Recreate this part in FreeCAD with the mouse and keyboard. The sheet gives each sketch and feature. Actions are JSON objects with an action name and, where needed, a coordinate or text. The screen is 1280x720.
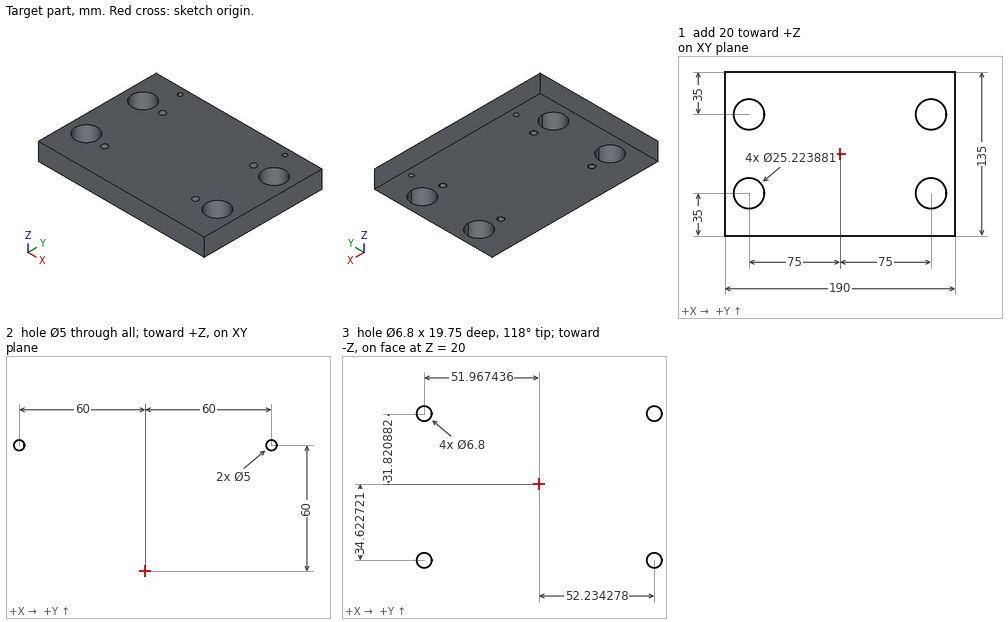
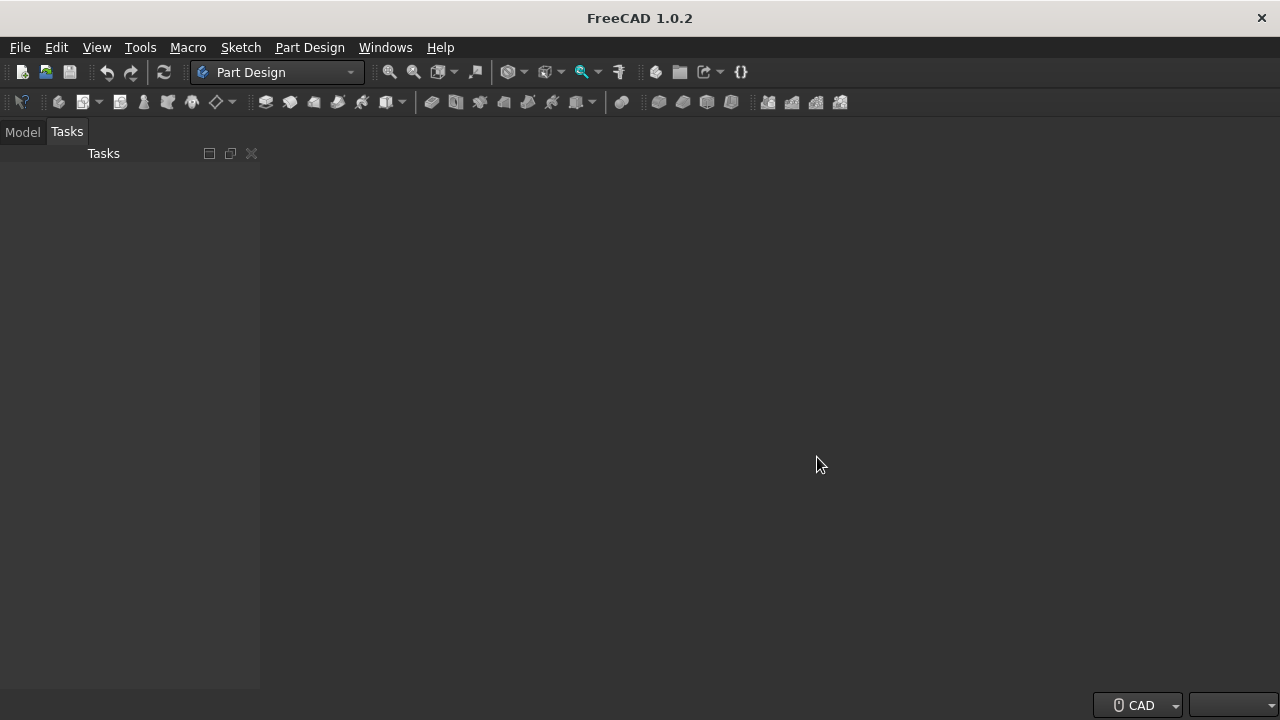
{"action": "left_click", "coordinate": [22, 72]}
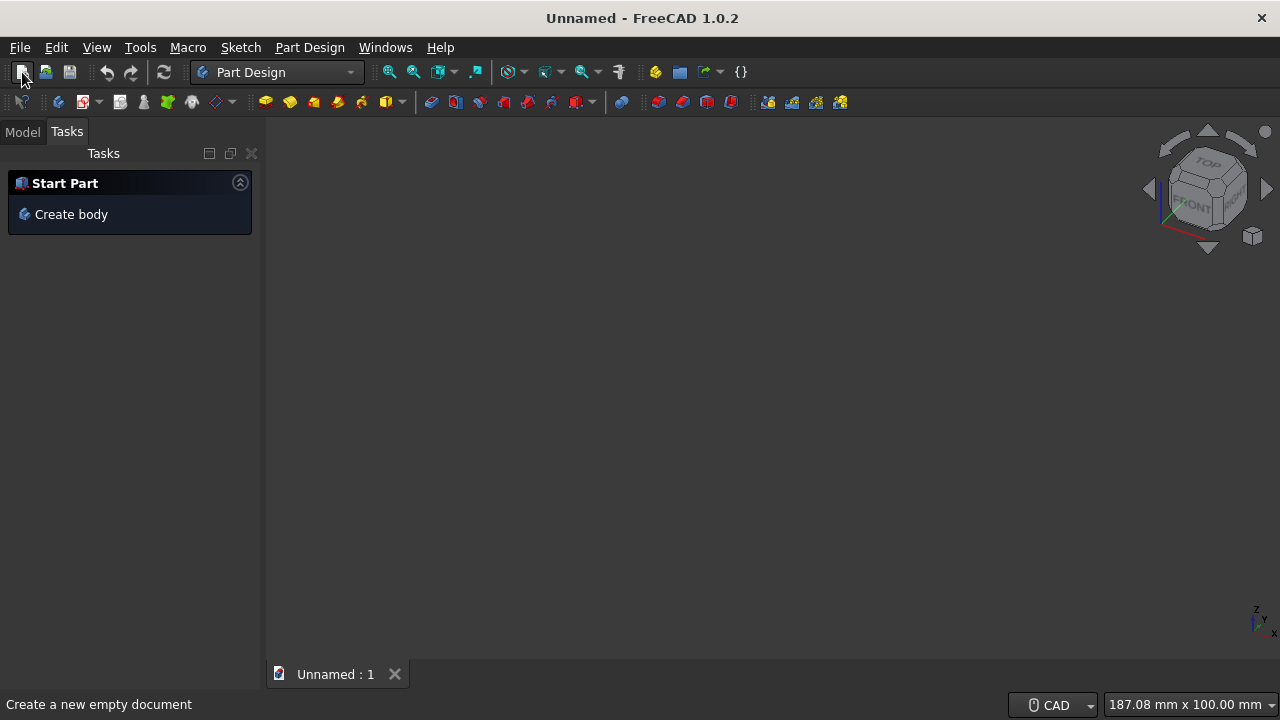
{"action": "left_click", "coordinate": [84, 102]}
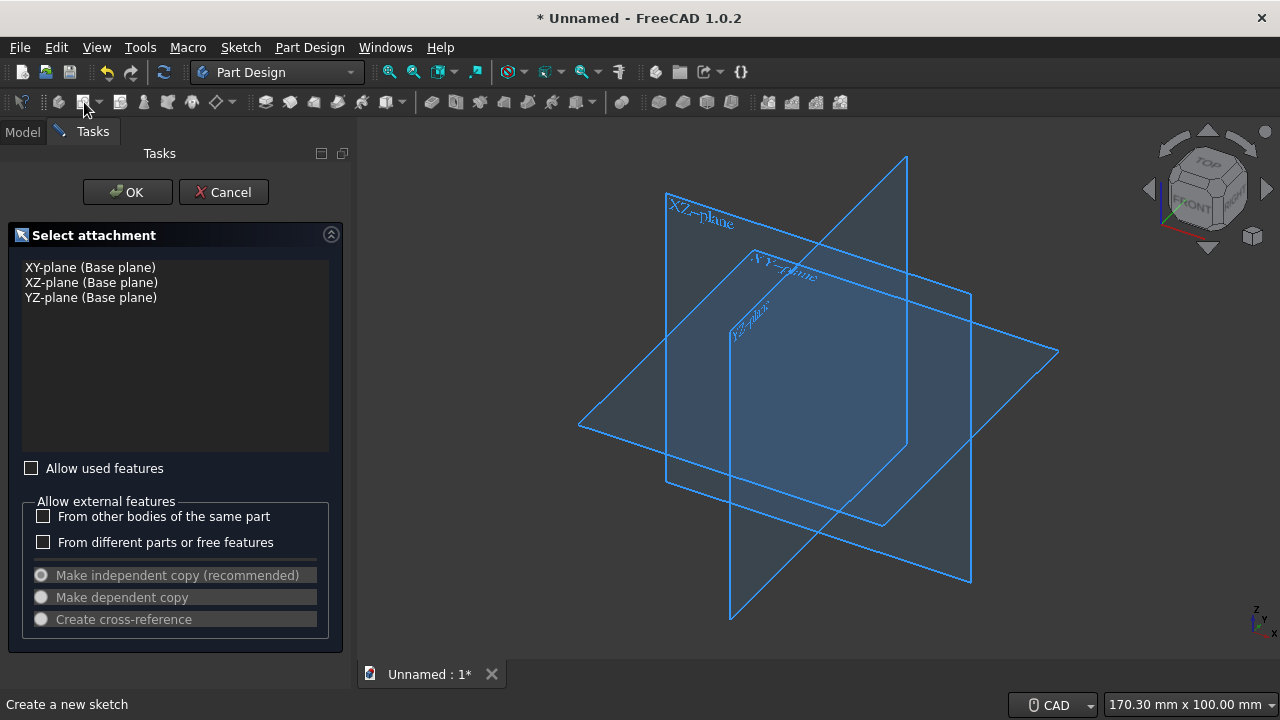
{"action": "left_click", "coordinate": [82, 268]}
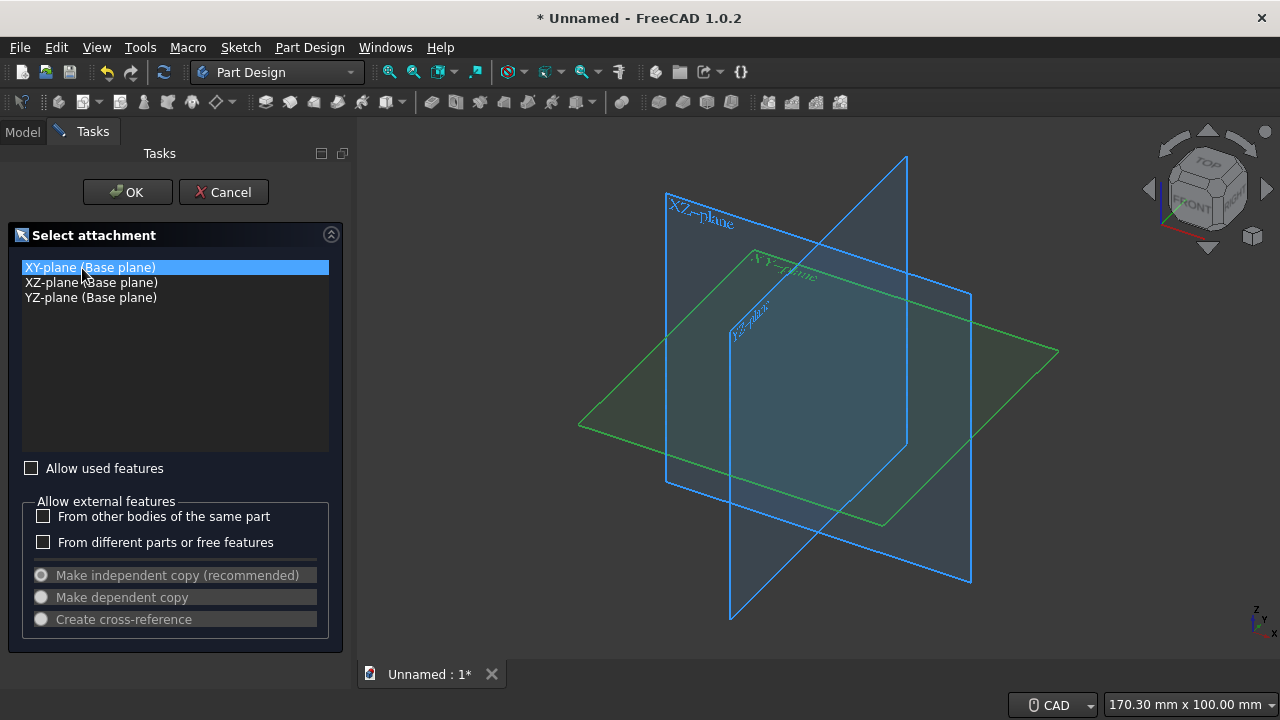
{"action": "left_click", "coordinate": [128, 192]}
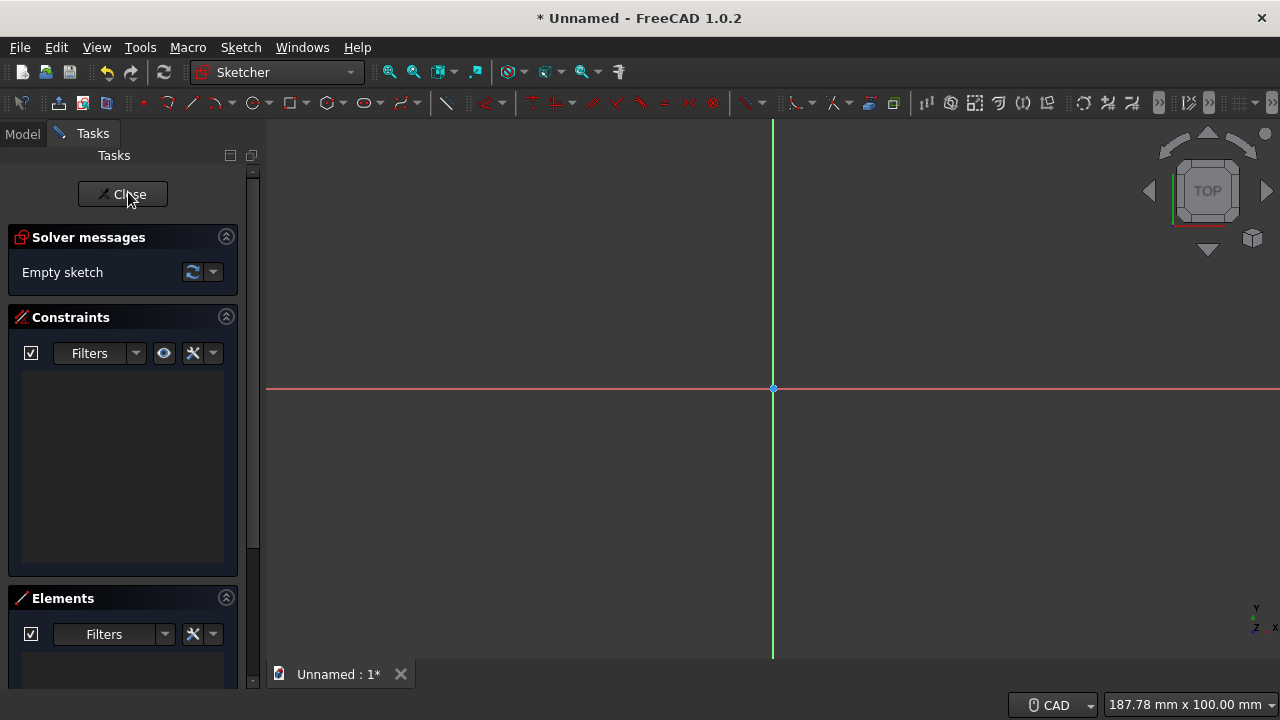
{"action": "scroll", "coordinate": [649, 389], "scroll_direction": "down", "scroll_amount": 4}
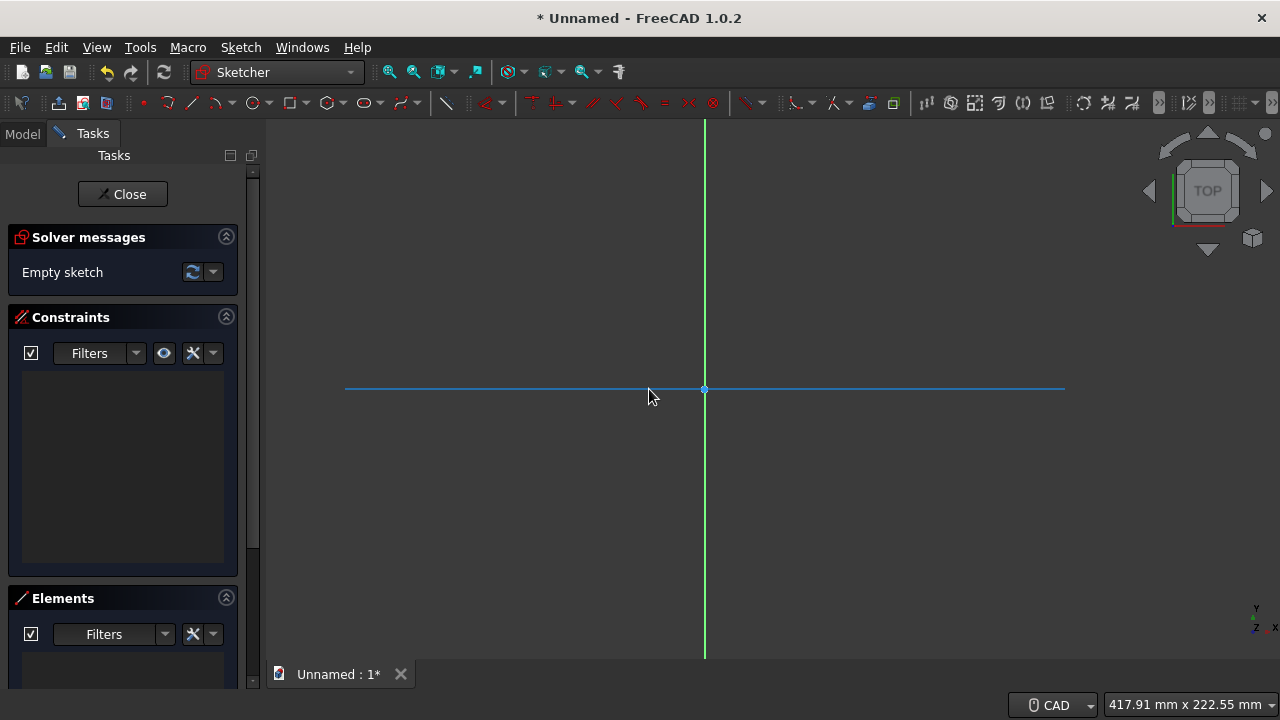
{"action": "left_click", "coordinate": [308, 104]}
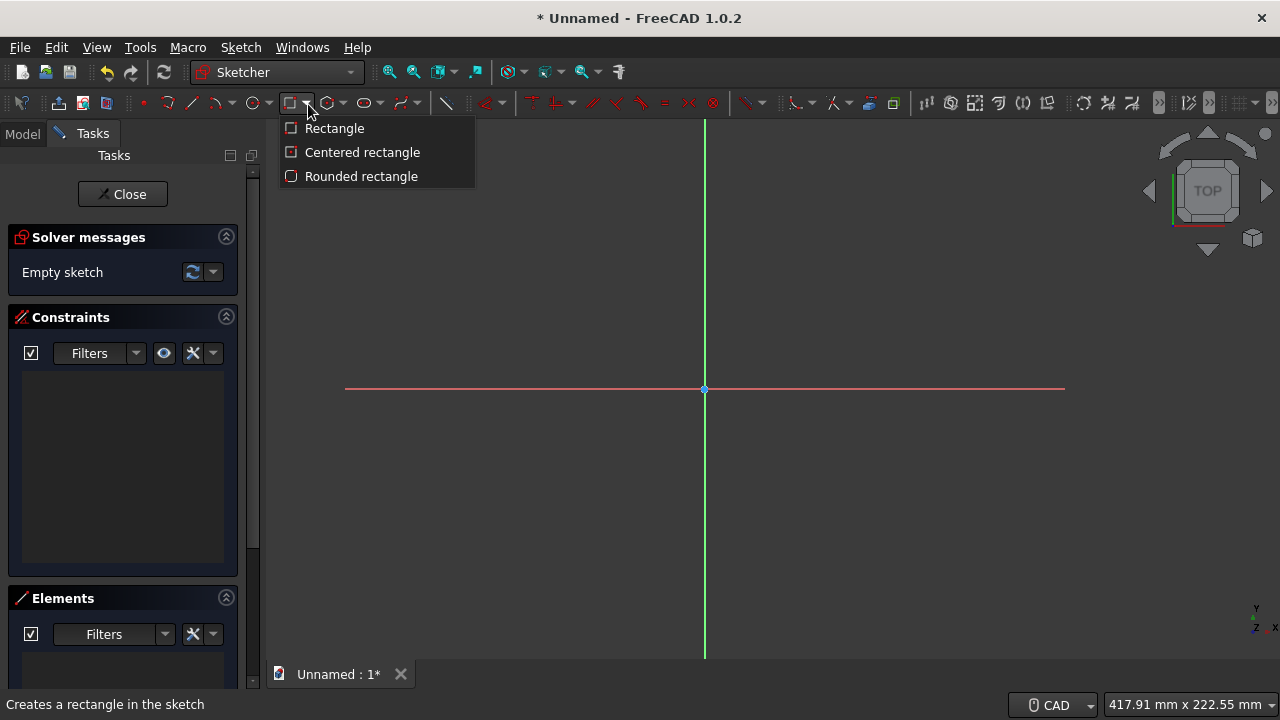
{"action": "left_click", "coordinate": [378, 152]}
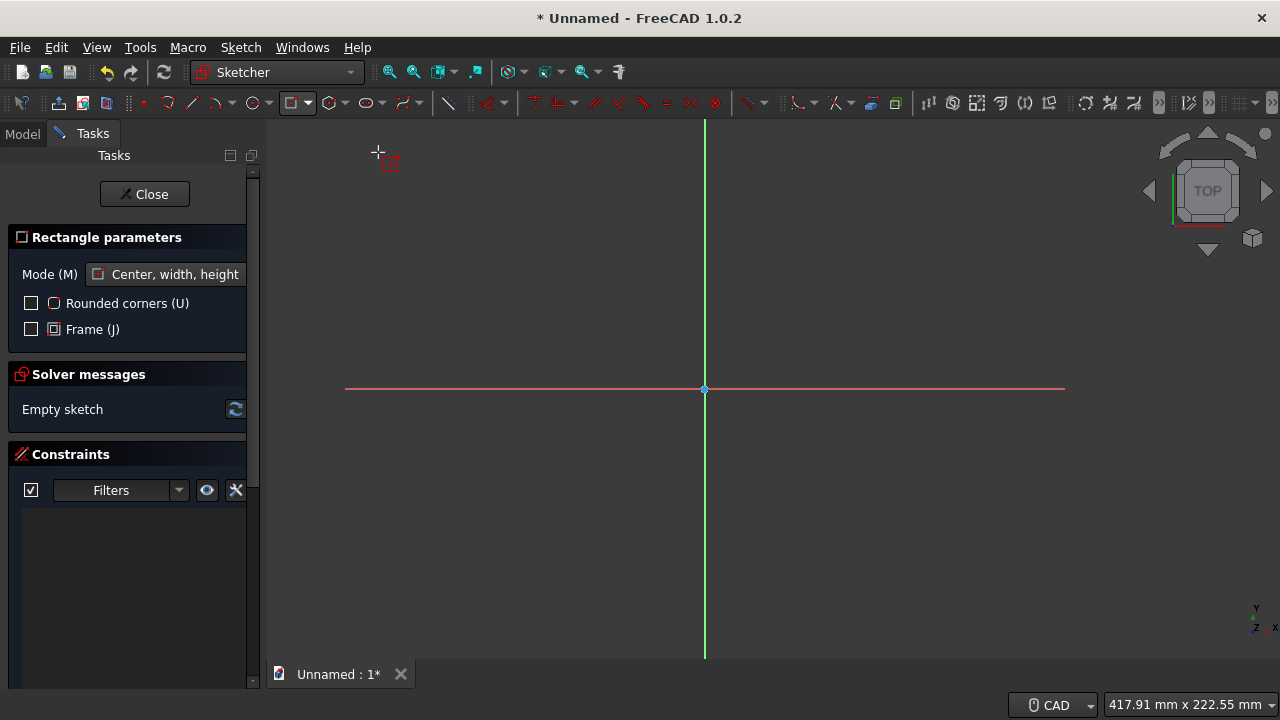
{"action": "left_click", "coordinate": [705, 389]}
{"action": "mouse_move", "coordinate": [935, 225]}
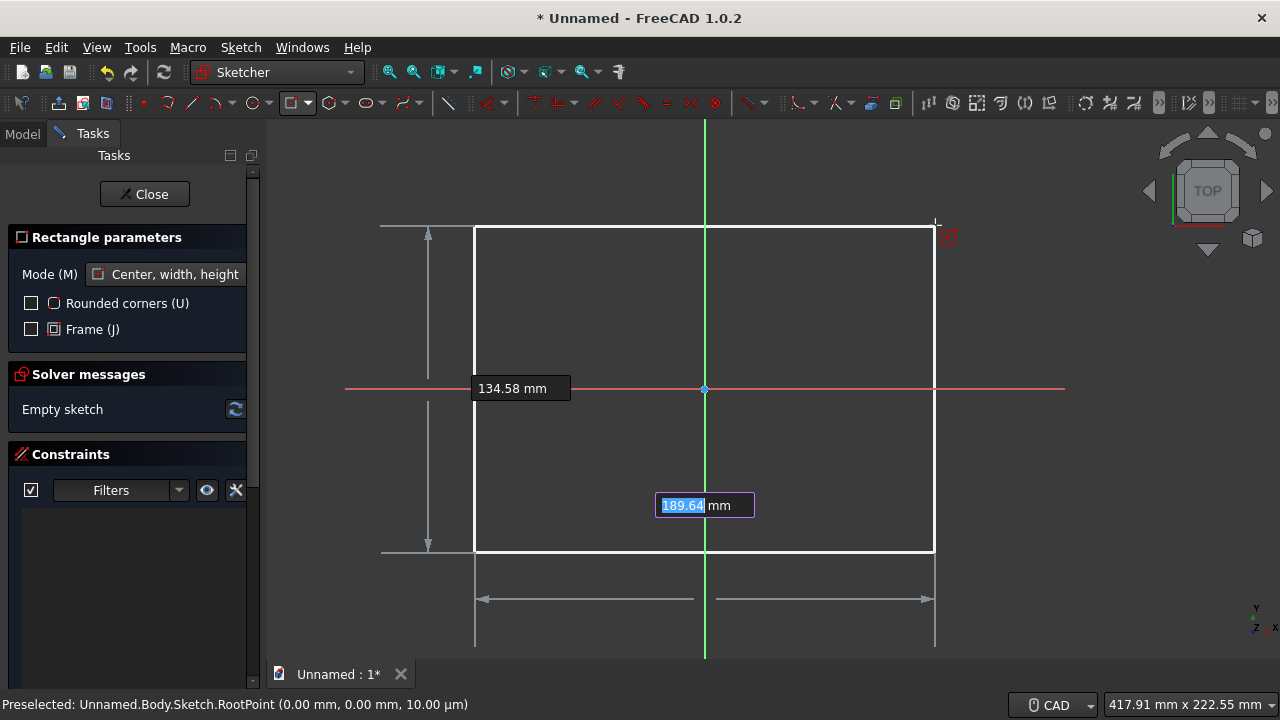
{"action": "type", "text": "190"}
{"action": "key", "text": "Tab"}
{"action": "type", "text": "135"}
{"action": "key", "text": "Return"}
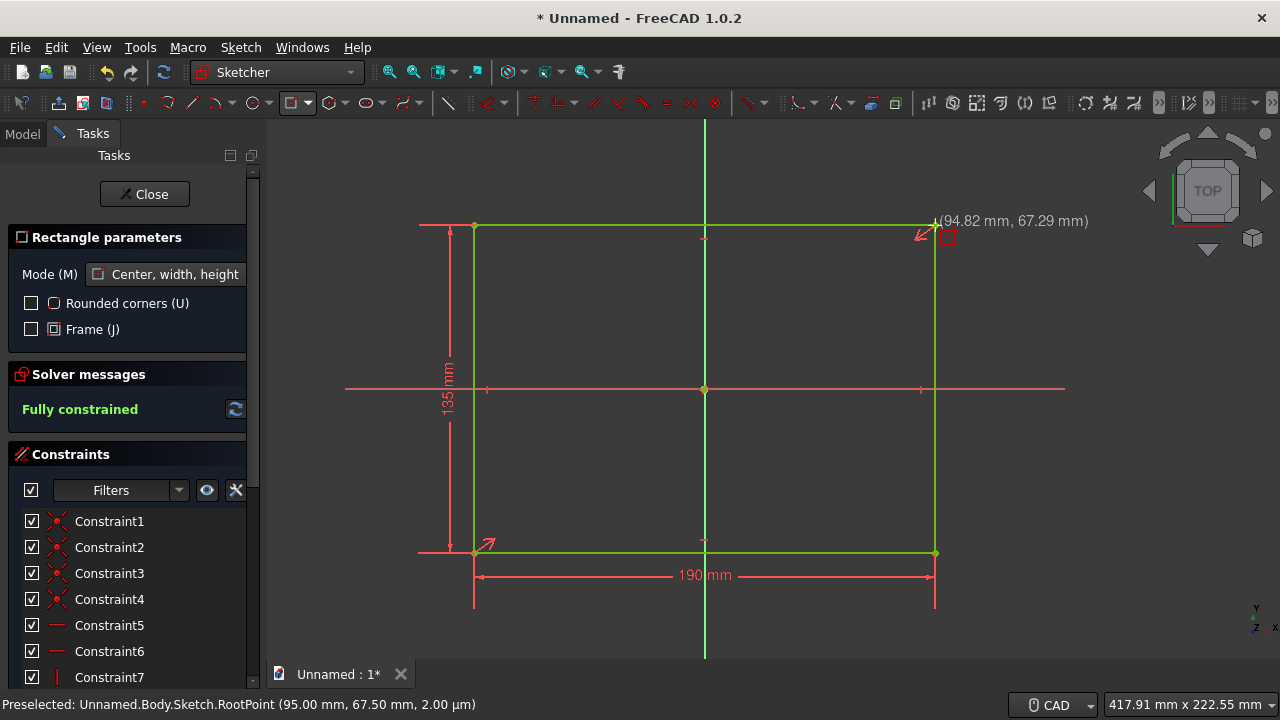
{"action": "left_click", "coordinate": [254, 104]}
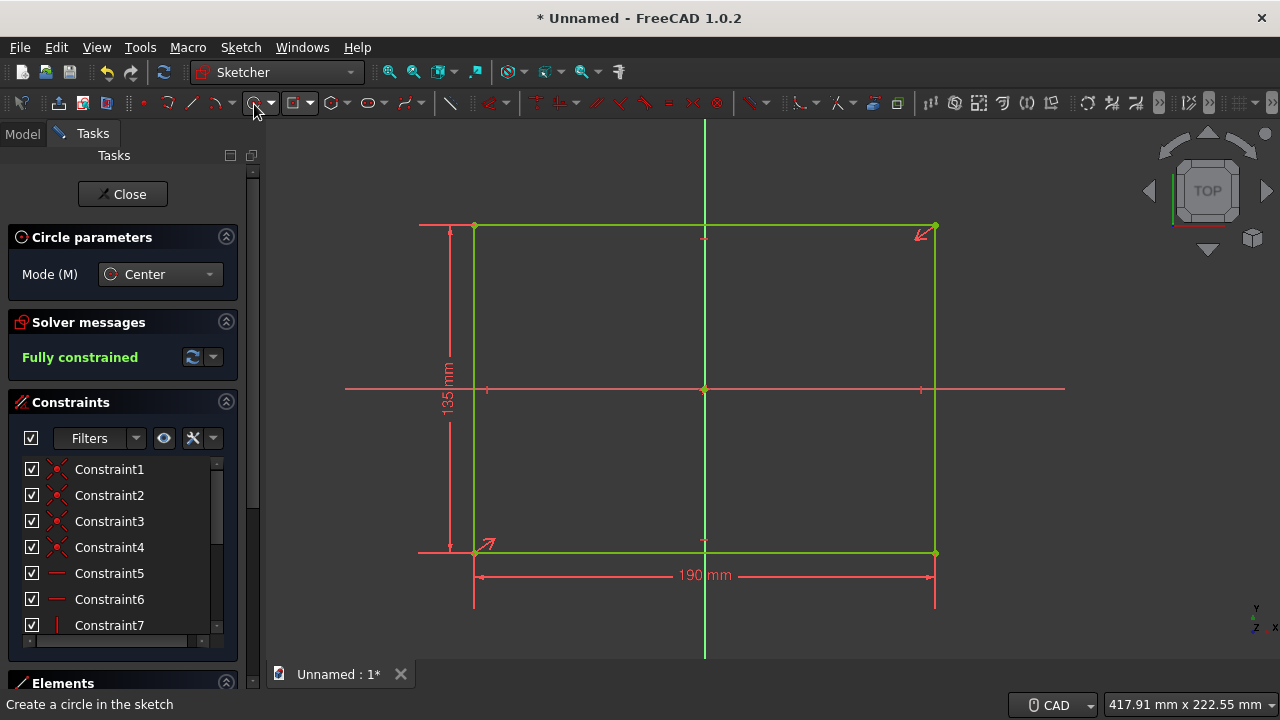
{"action": "left_click", "coordinate": [523, 468]}
{"action": "mouse_move", "coordinate": [545, 446]}